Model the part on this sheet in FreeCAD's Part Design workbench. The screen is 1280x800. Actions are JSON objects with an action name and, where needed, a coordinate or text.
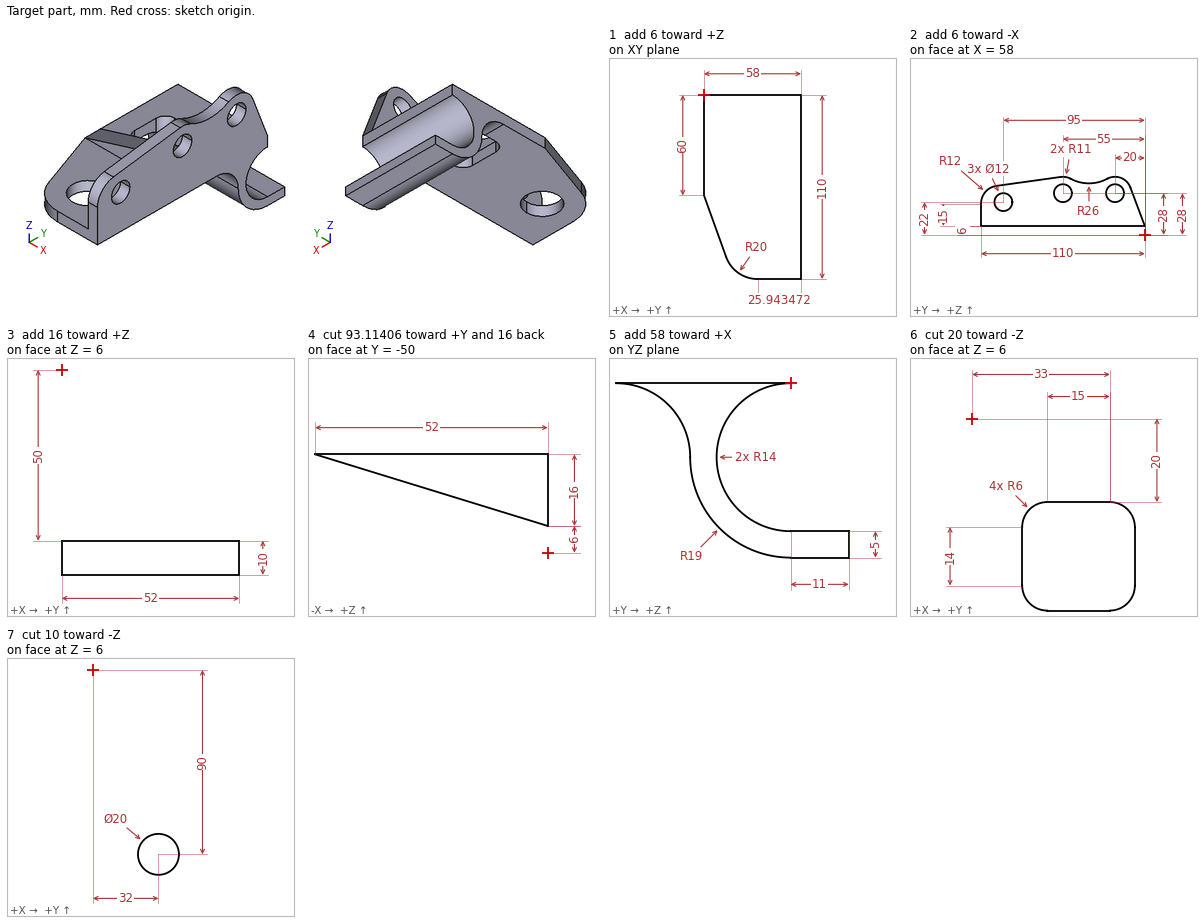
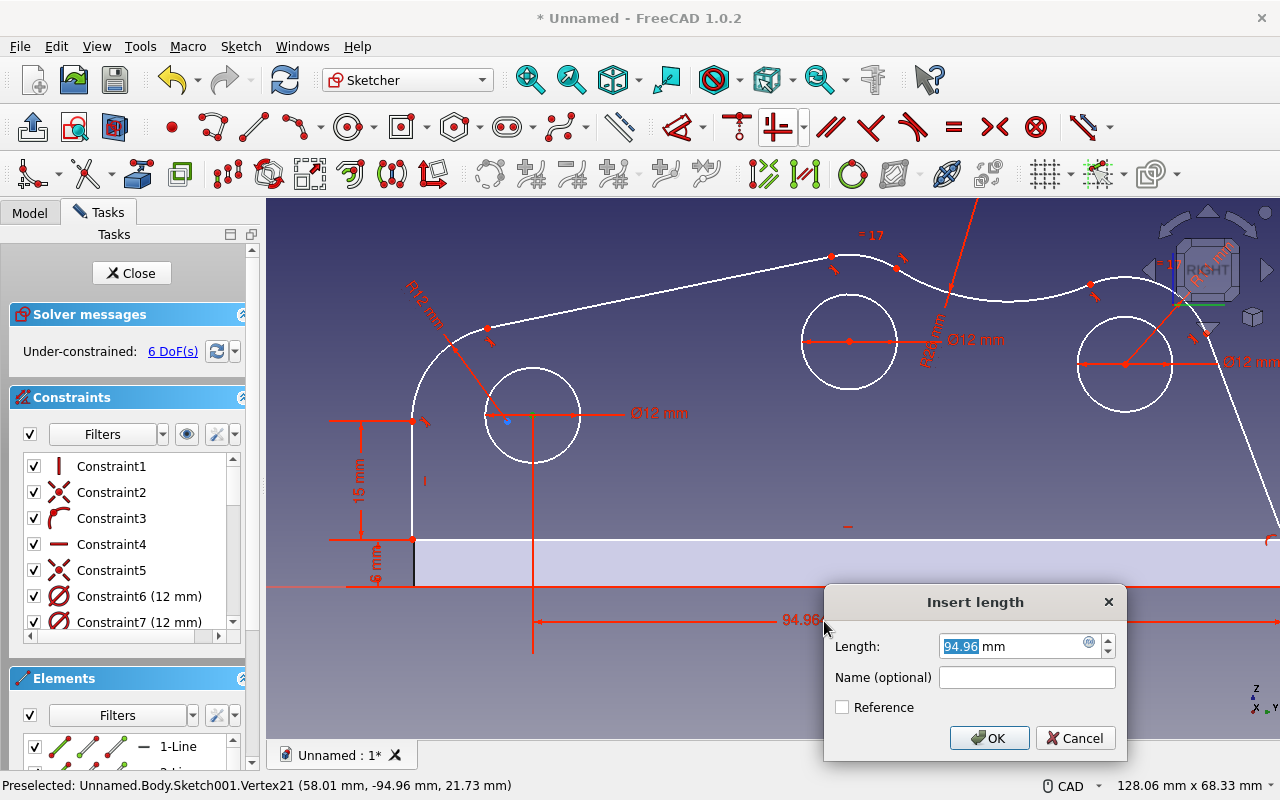
{"action": "type", "text": "95"}
{"action": "key", "text": "Return"}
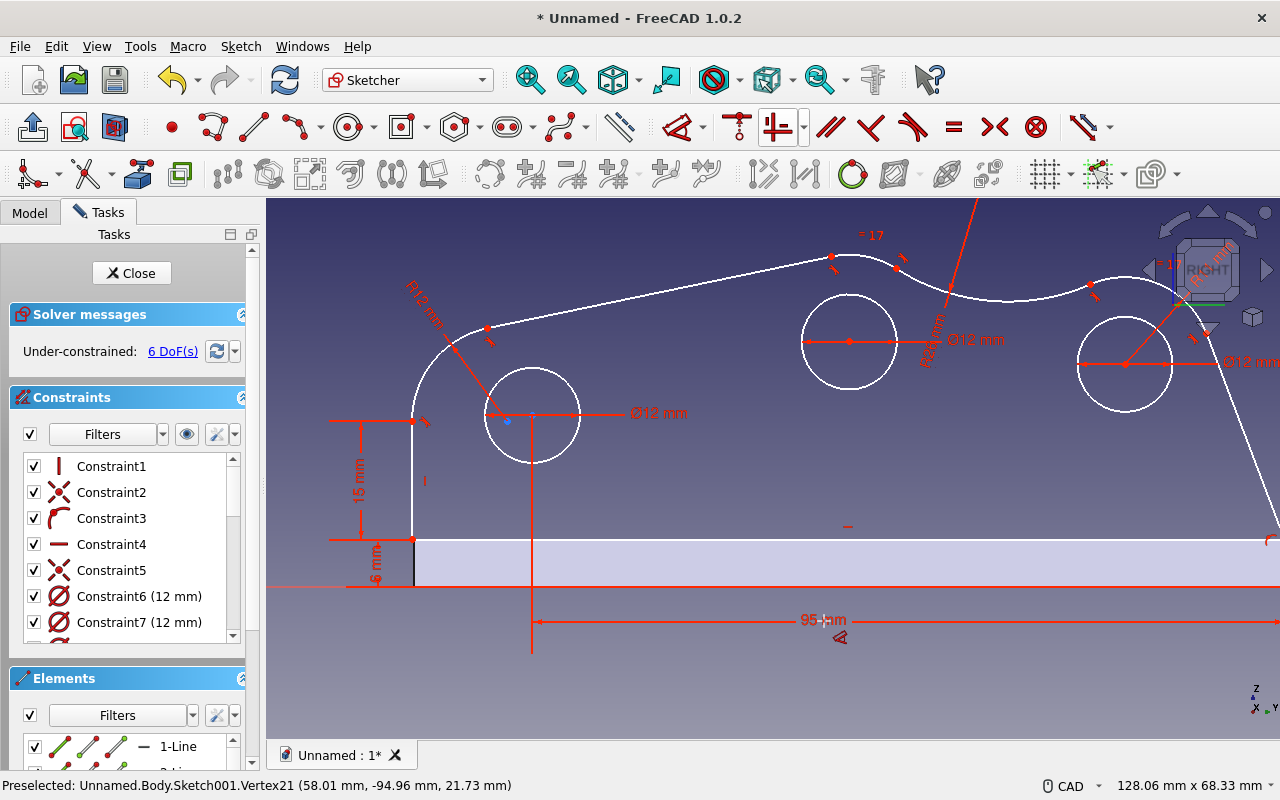
{"action": "left_click", "coordinate": [532, 415]}
{"action": "left_click", "coordinate": [498, 501]}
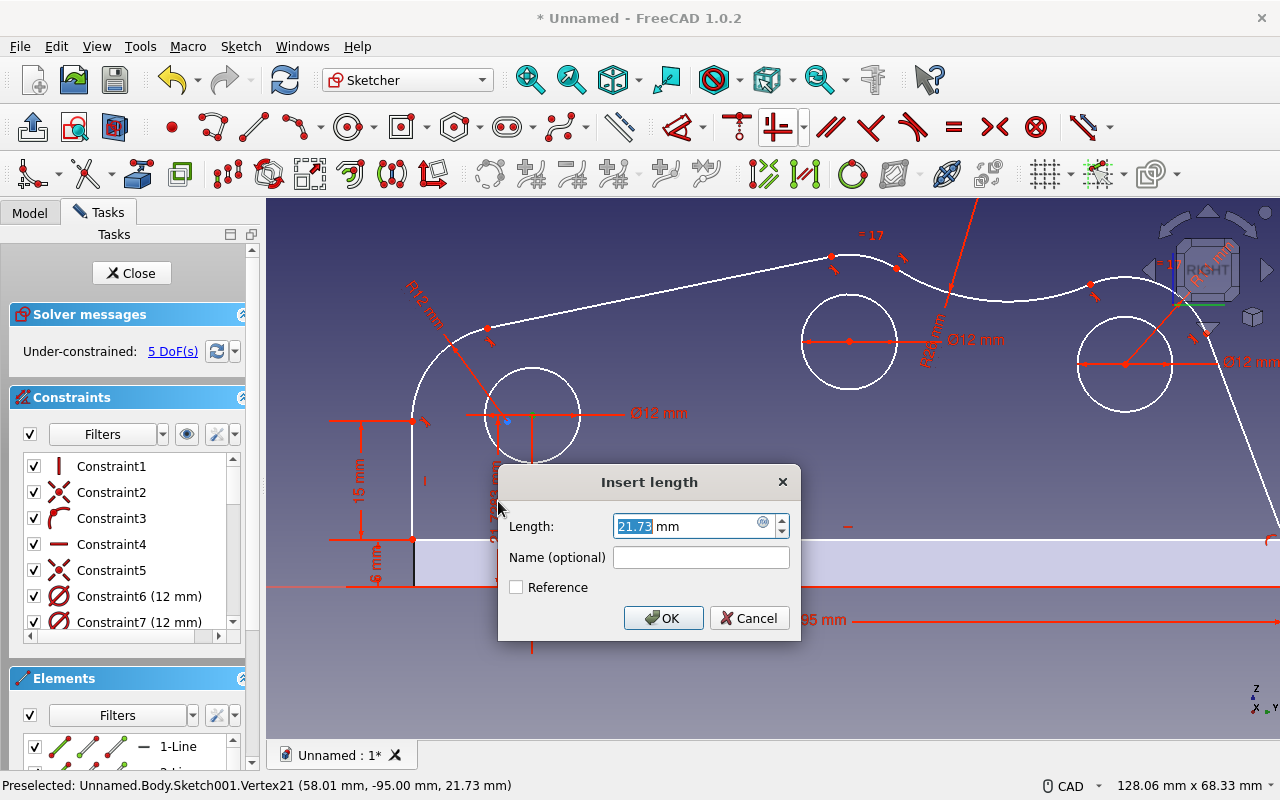
{"action": "type", "text": "22"}
{"action": "key", "text": "Return"}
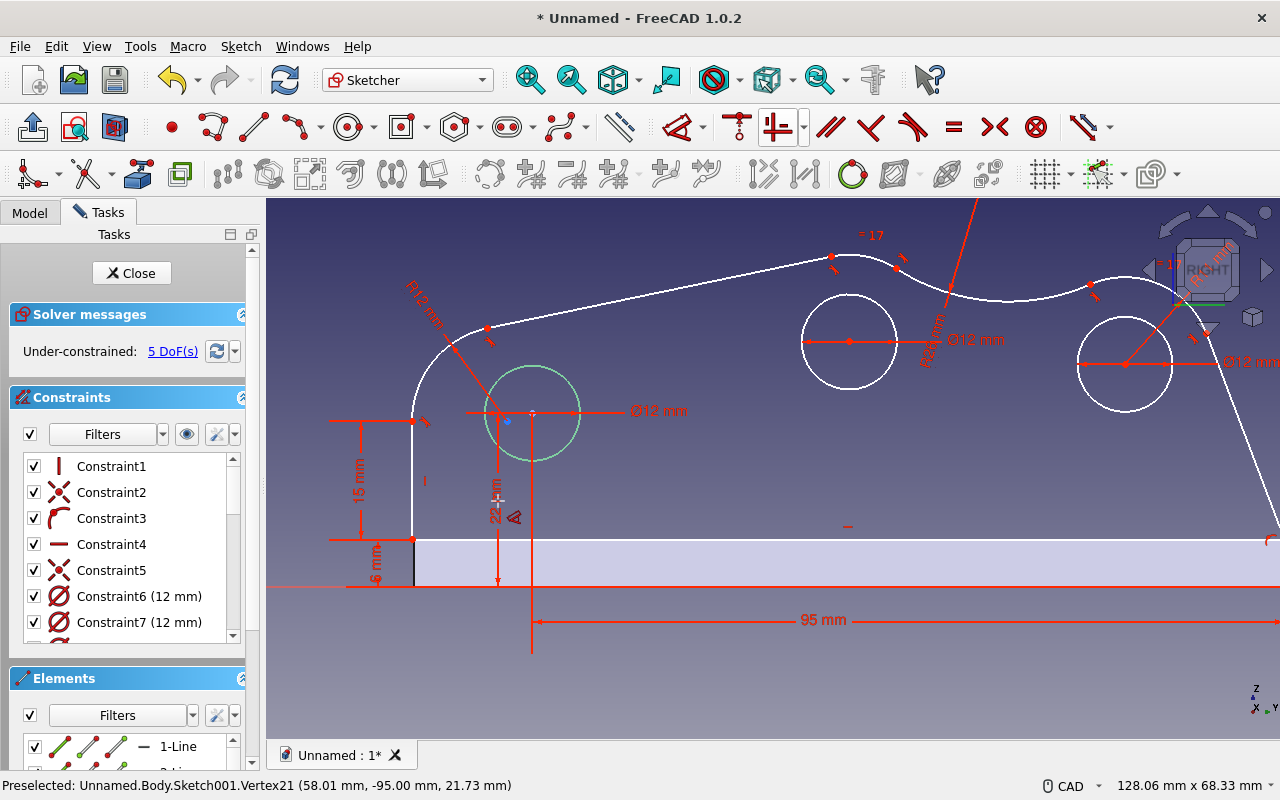
{"action": "left_click", "coordinate": [849, 342]}
{"action": "left_click", "coordinate": [982, 621]}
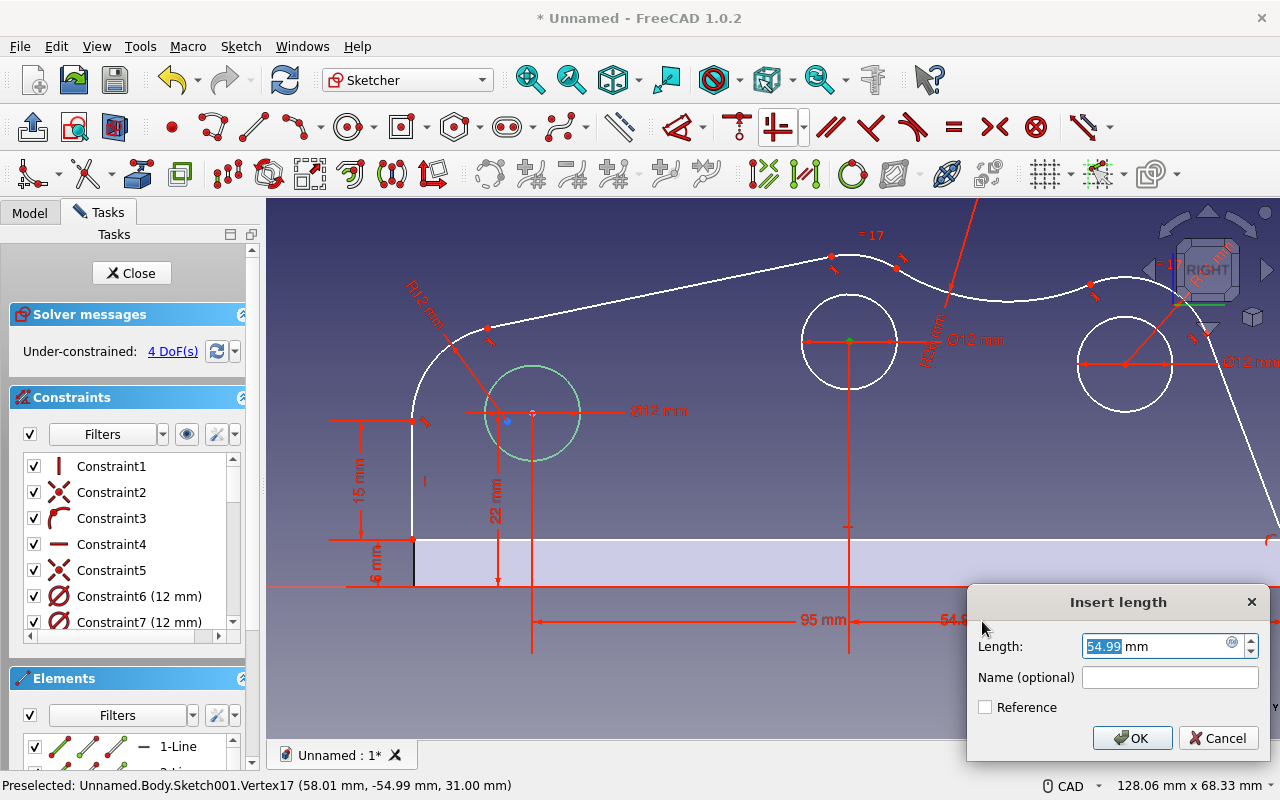
{"action": "type", "text": "55"}
{"action": "key", "text": "Return"}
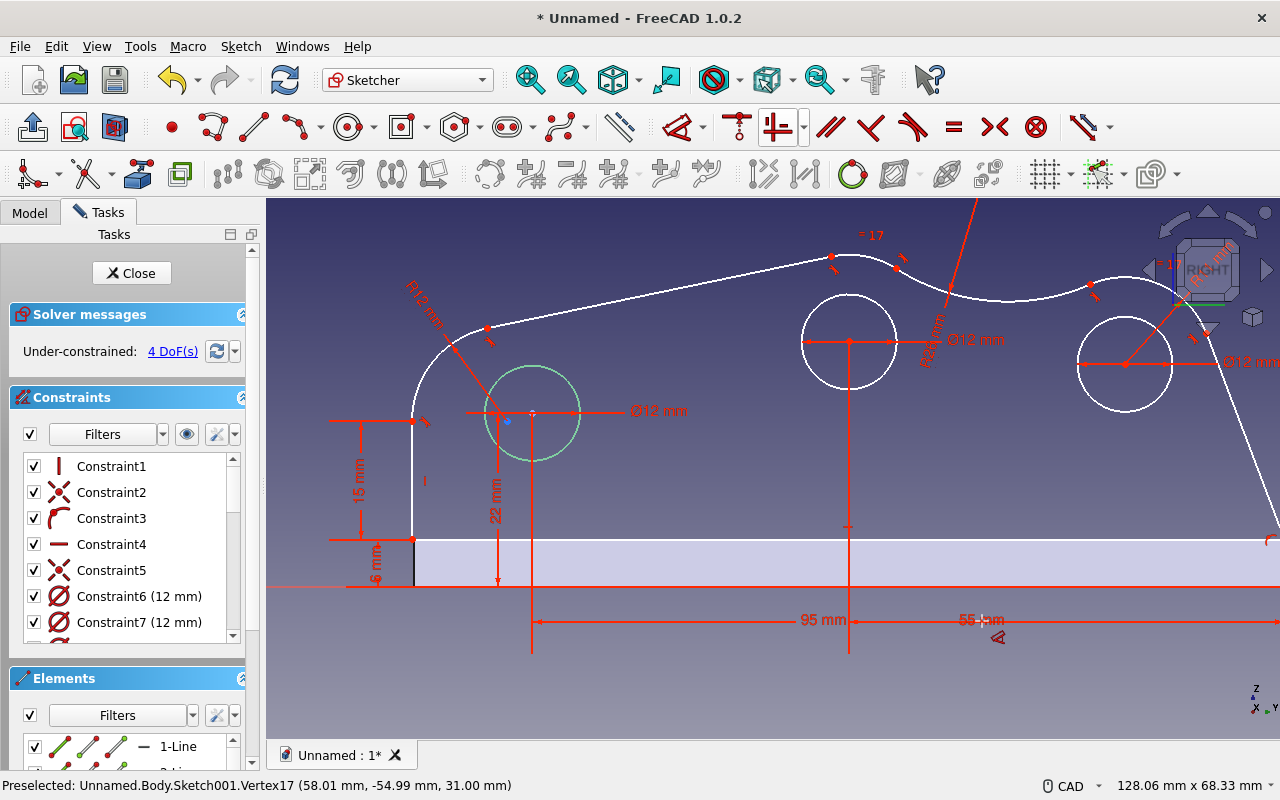
{"action": "left_click", "coordinate": [849, 342]}
{"action": "left_click", "coordinate": [815, 465]}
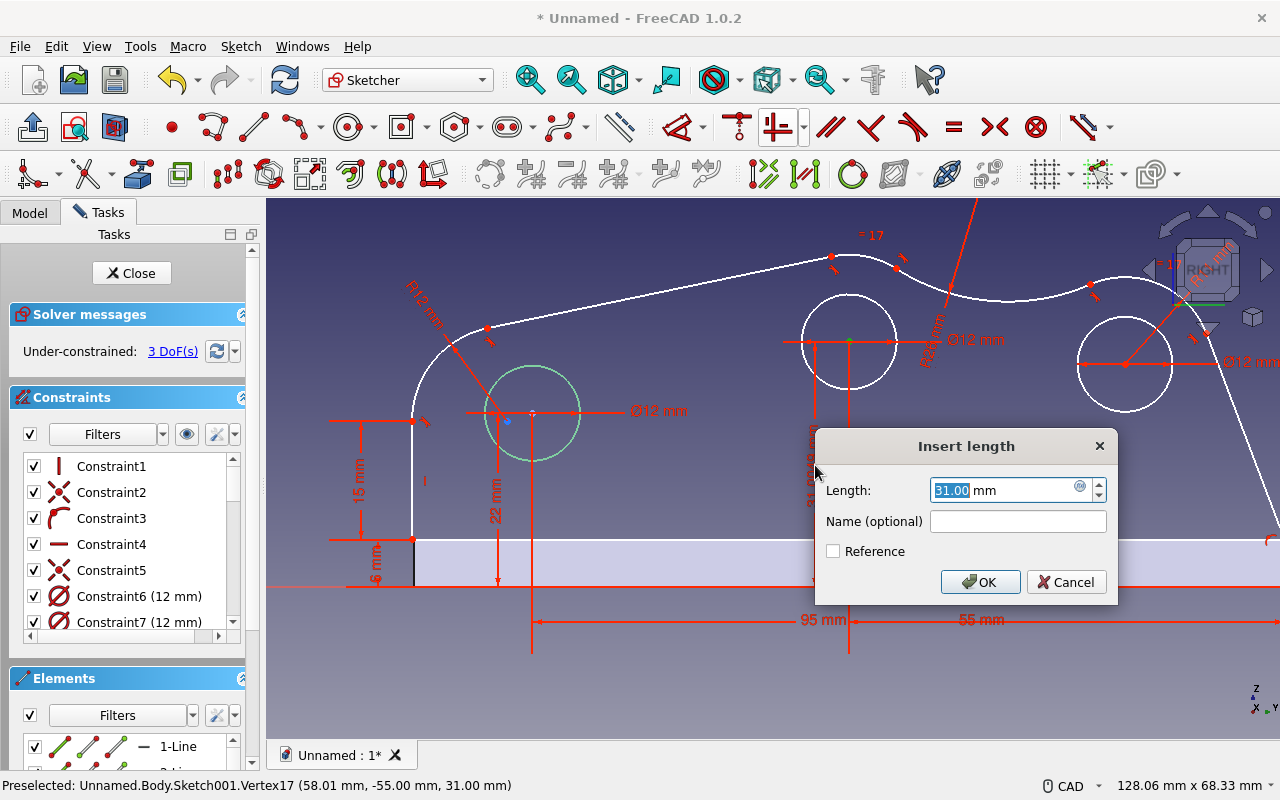
{"action": "type", "text": "28"}
{"action": "key", "text": "Return"}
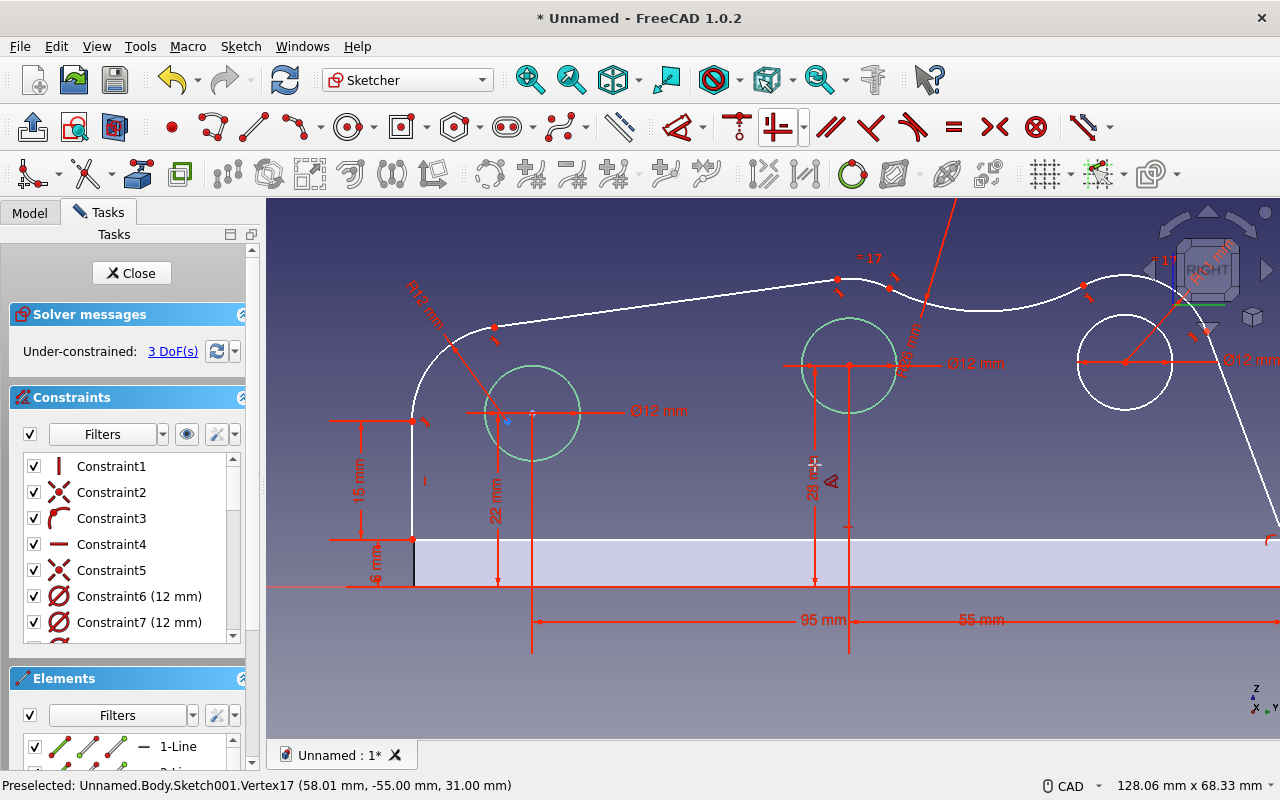
{"action": "scroll", "coordinate": [410, 540], "scroll_direction": "down", "scroll_amount": 2}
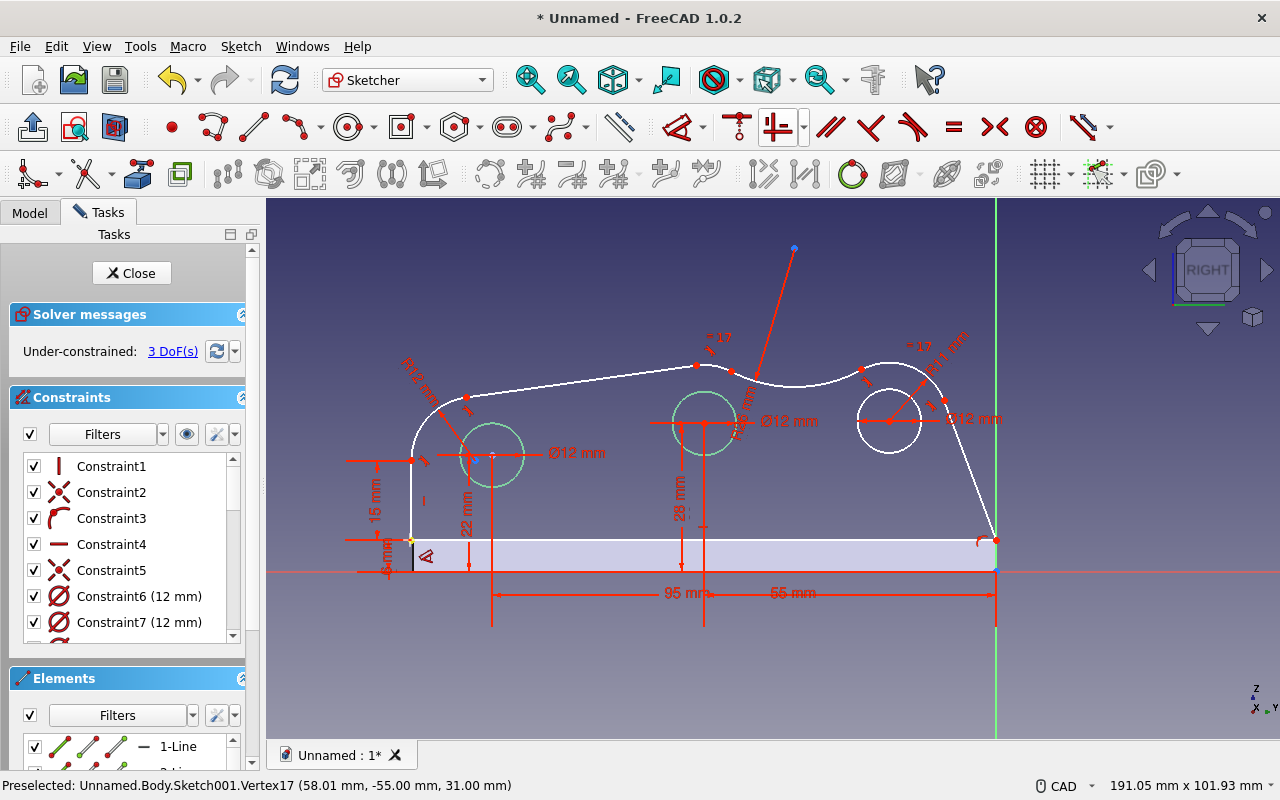
{"action": "left_click", "coordinate": [889, 421]}
{"action": "left_click", "coordinate": [943, 606]}